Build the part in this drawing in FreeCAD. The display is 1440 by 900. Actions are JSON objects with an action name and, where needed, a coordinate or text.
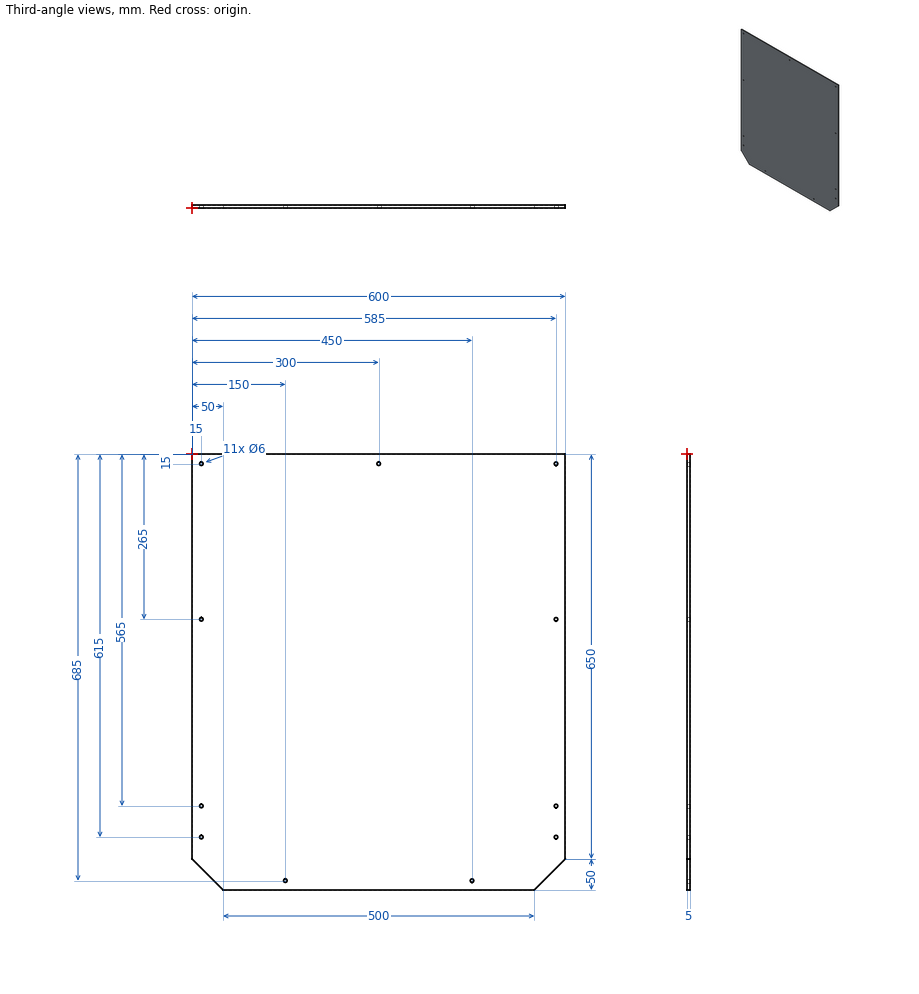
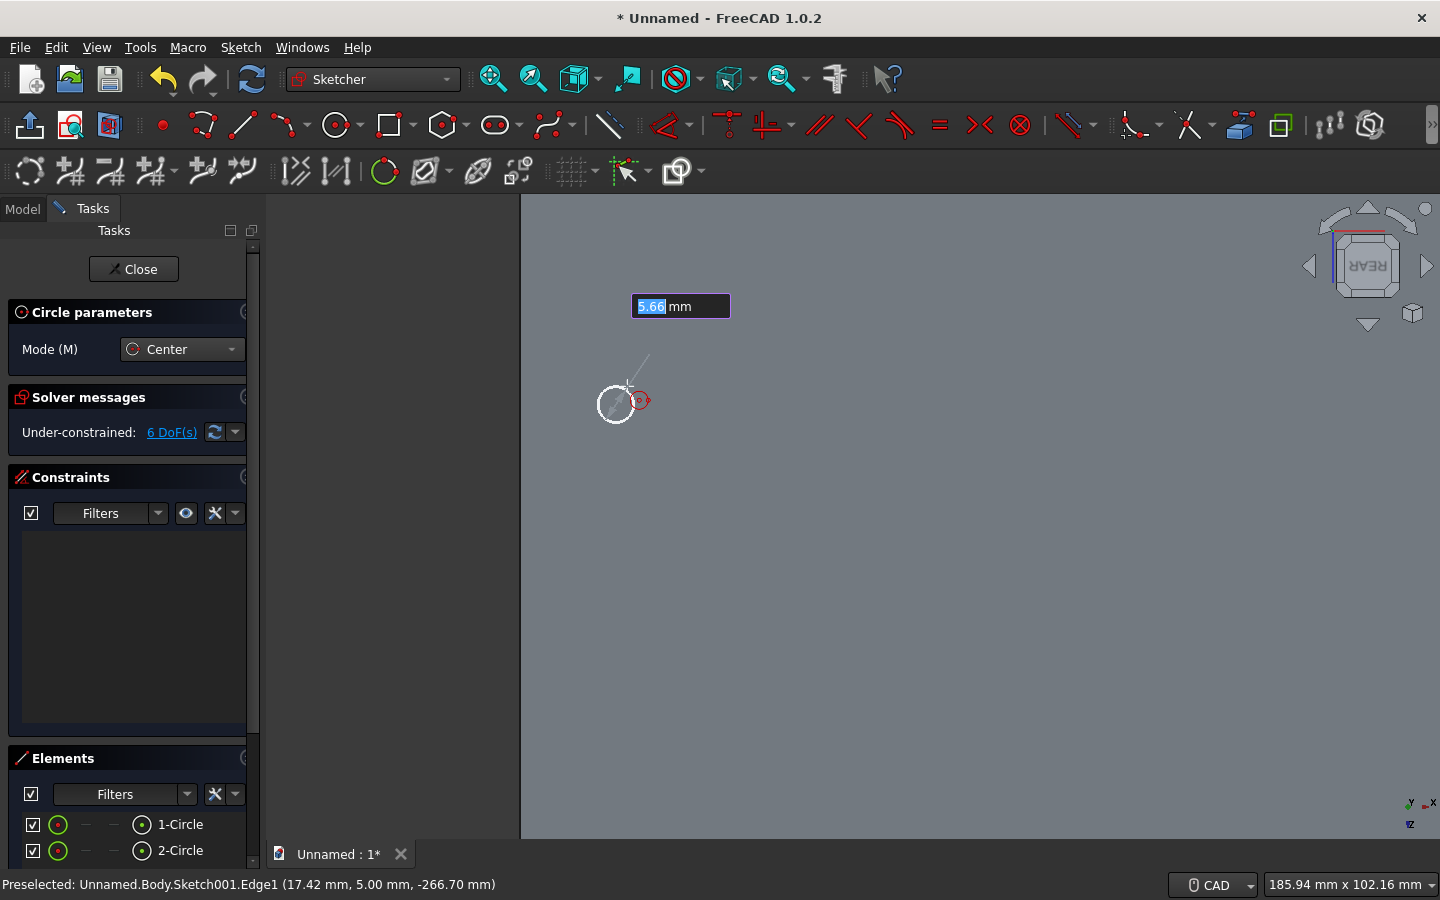
{"action": "left_click", "coordinate": [628, 387]}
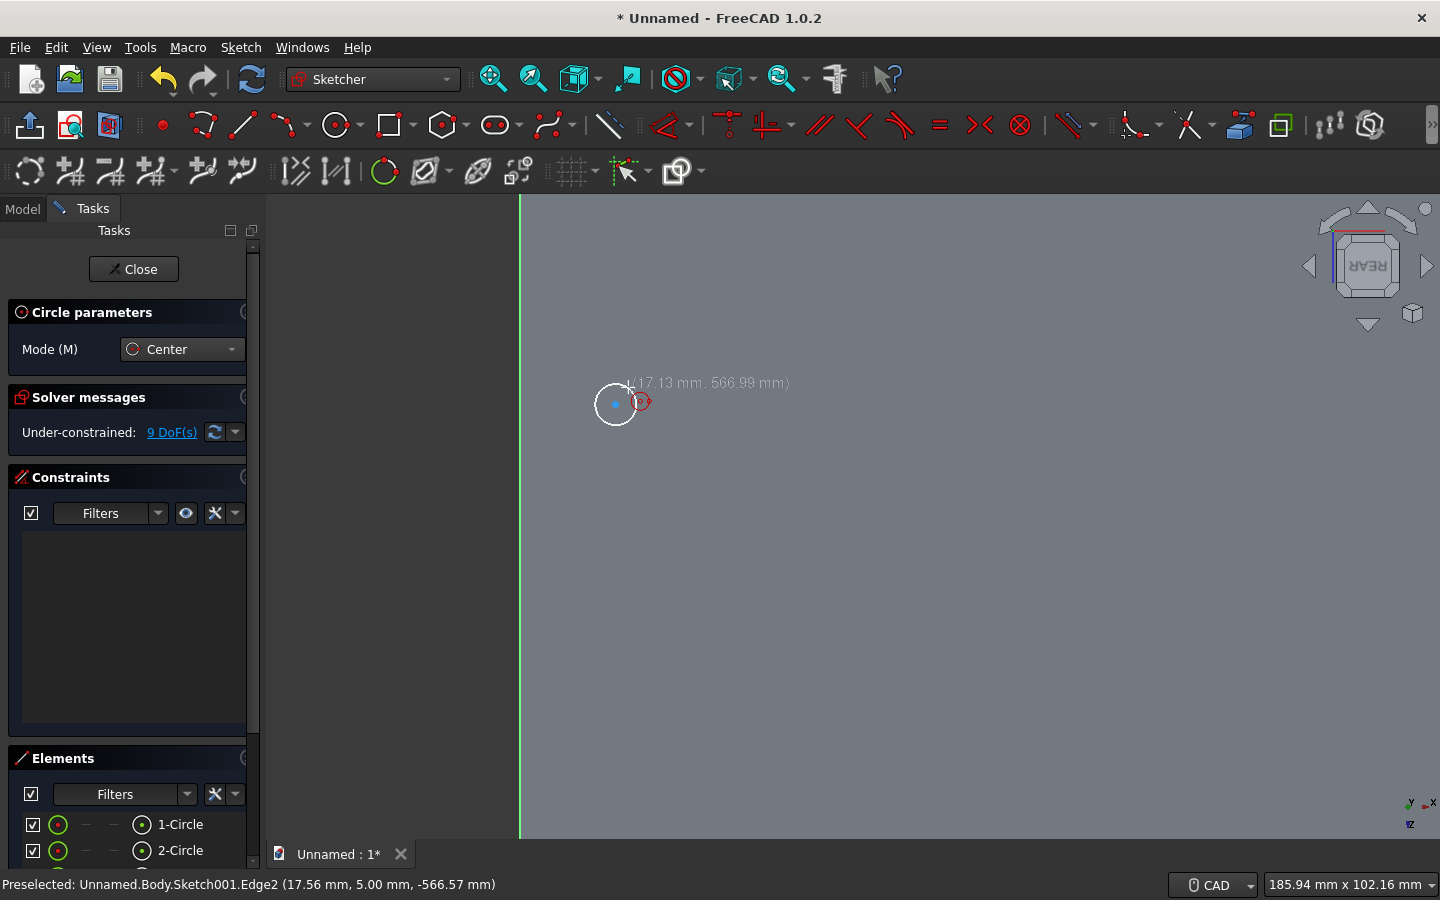
{"action": "scroll", "coordinate": [626, 389], "scroll_direction": "down", "scroll_amount": 12}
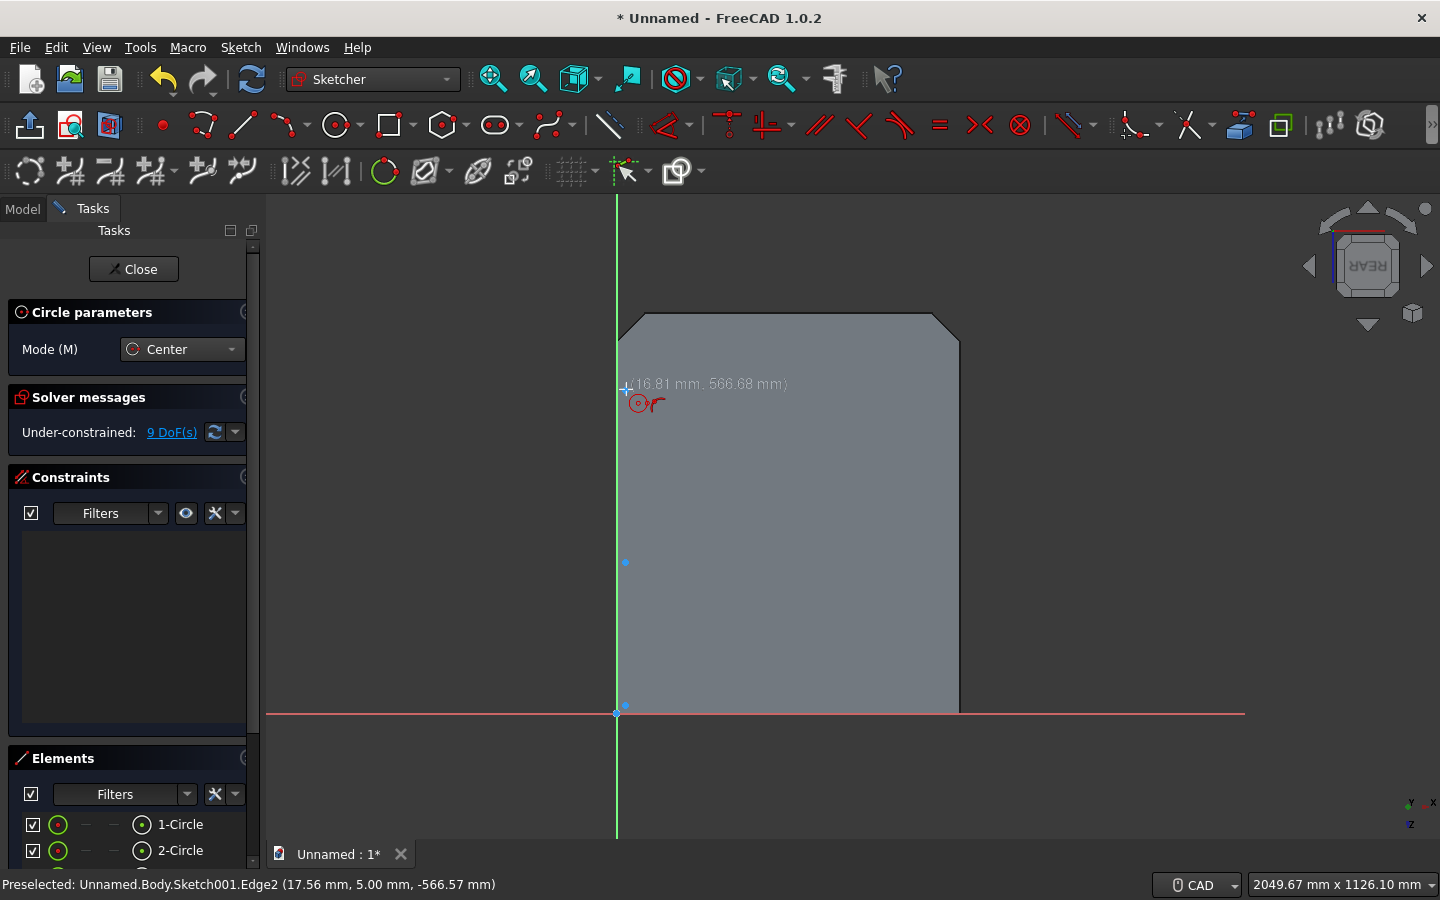
{"action": "scroll", "coordinate": [625, 362], "scroll_direction": "up", "scroll_amount": 13}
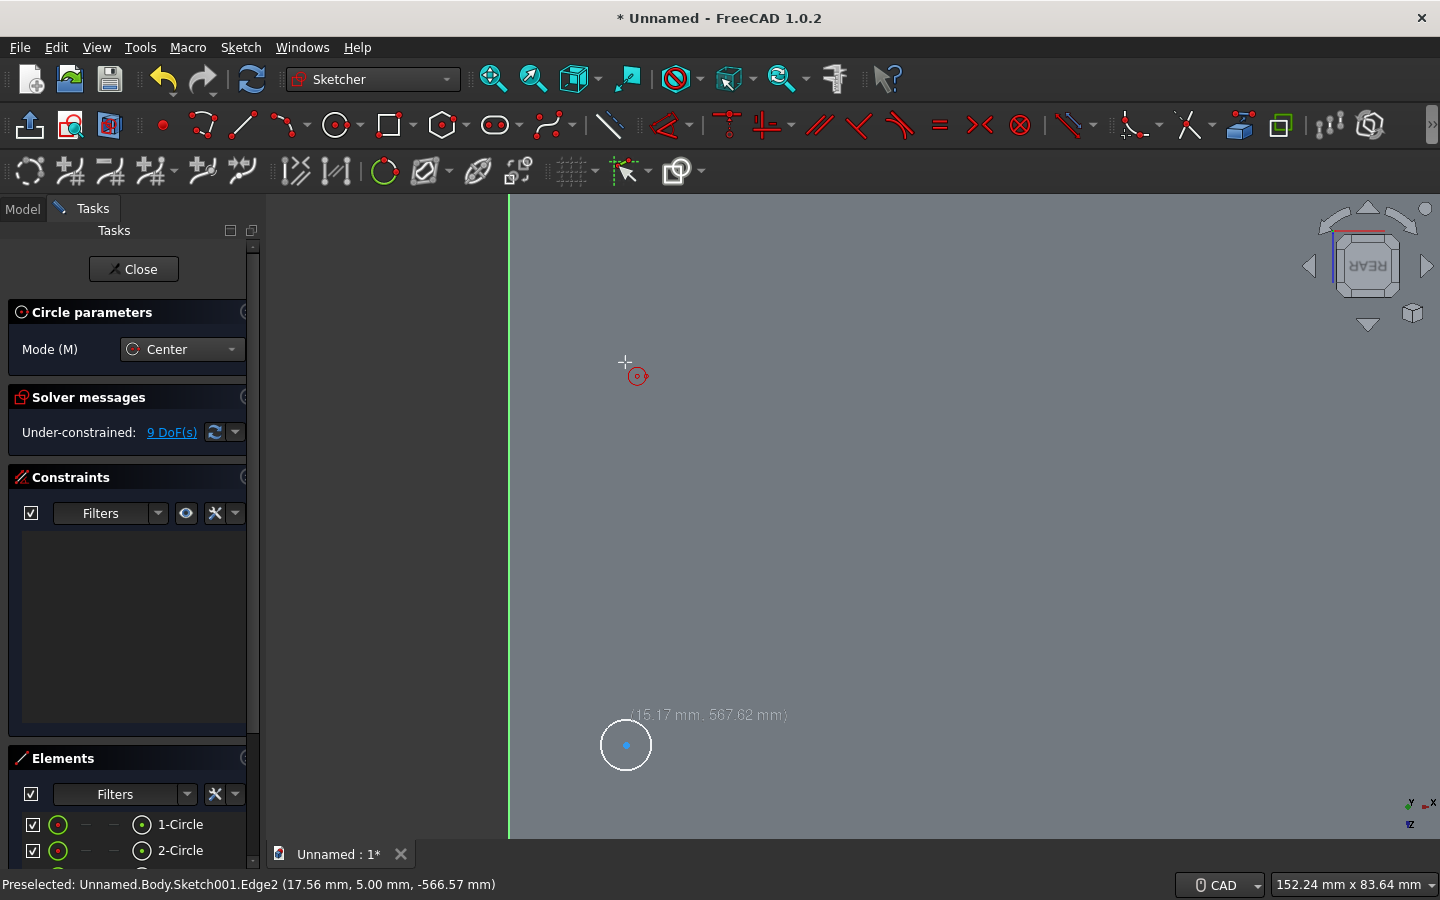
{"action": "scroll", "coordinate": [625, 362], "scroll_direction": "down", "scroll_amount": 13}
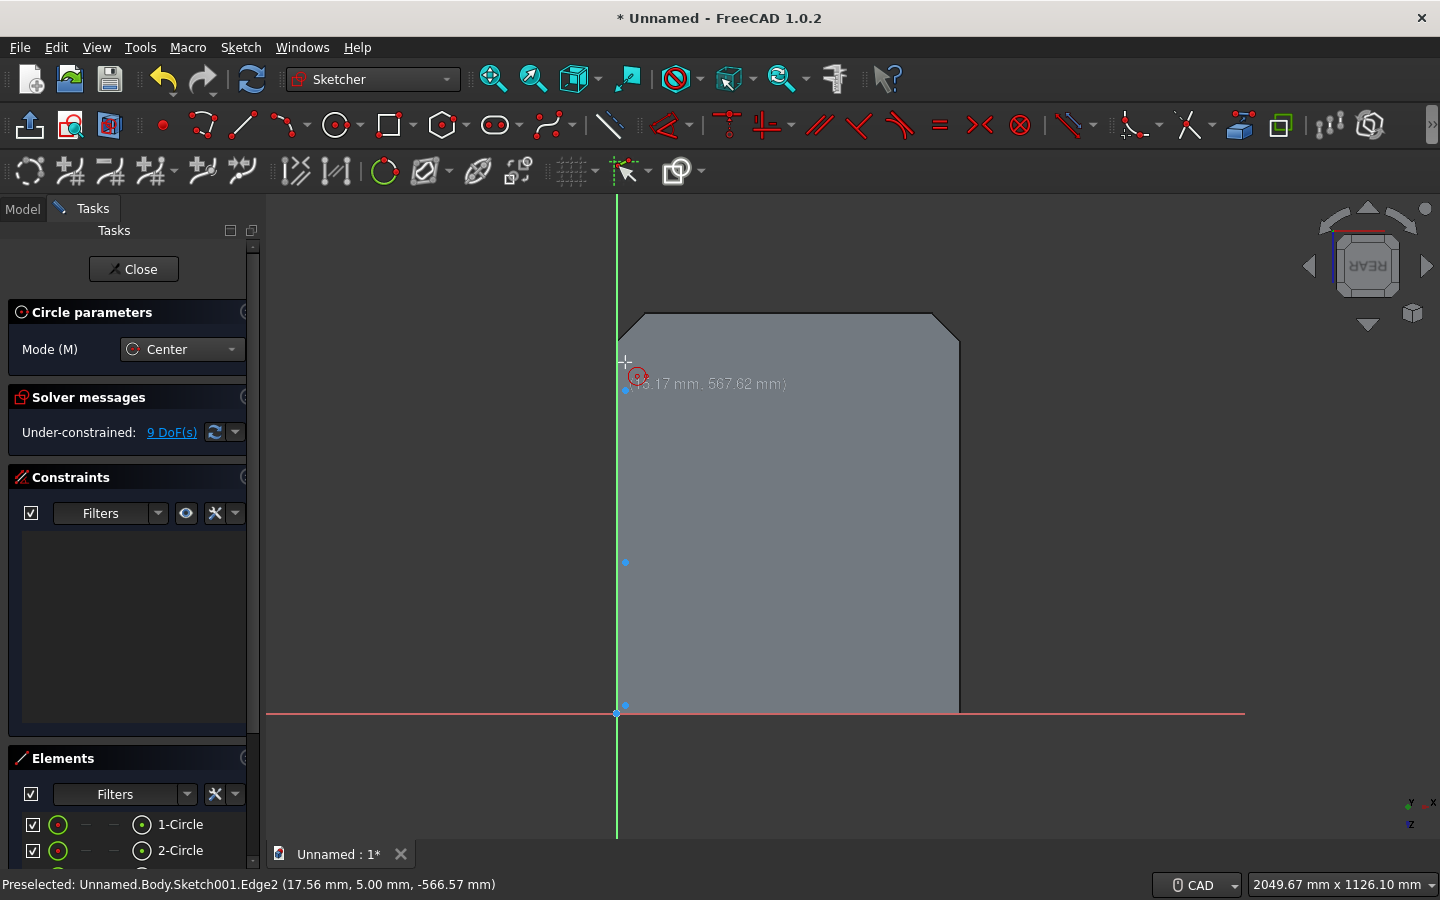
{"action": "scroll", "coordinate": [625, 362], "scroll_direction": "up", "scroll_amount": 4}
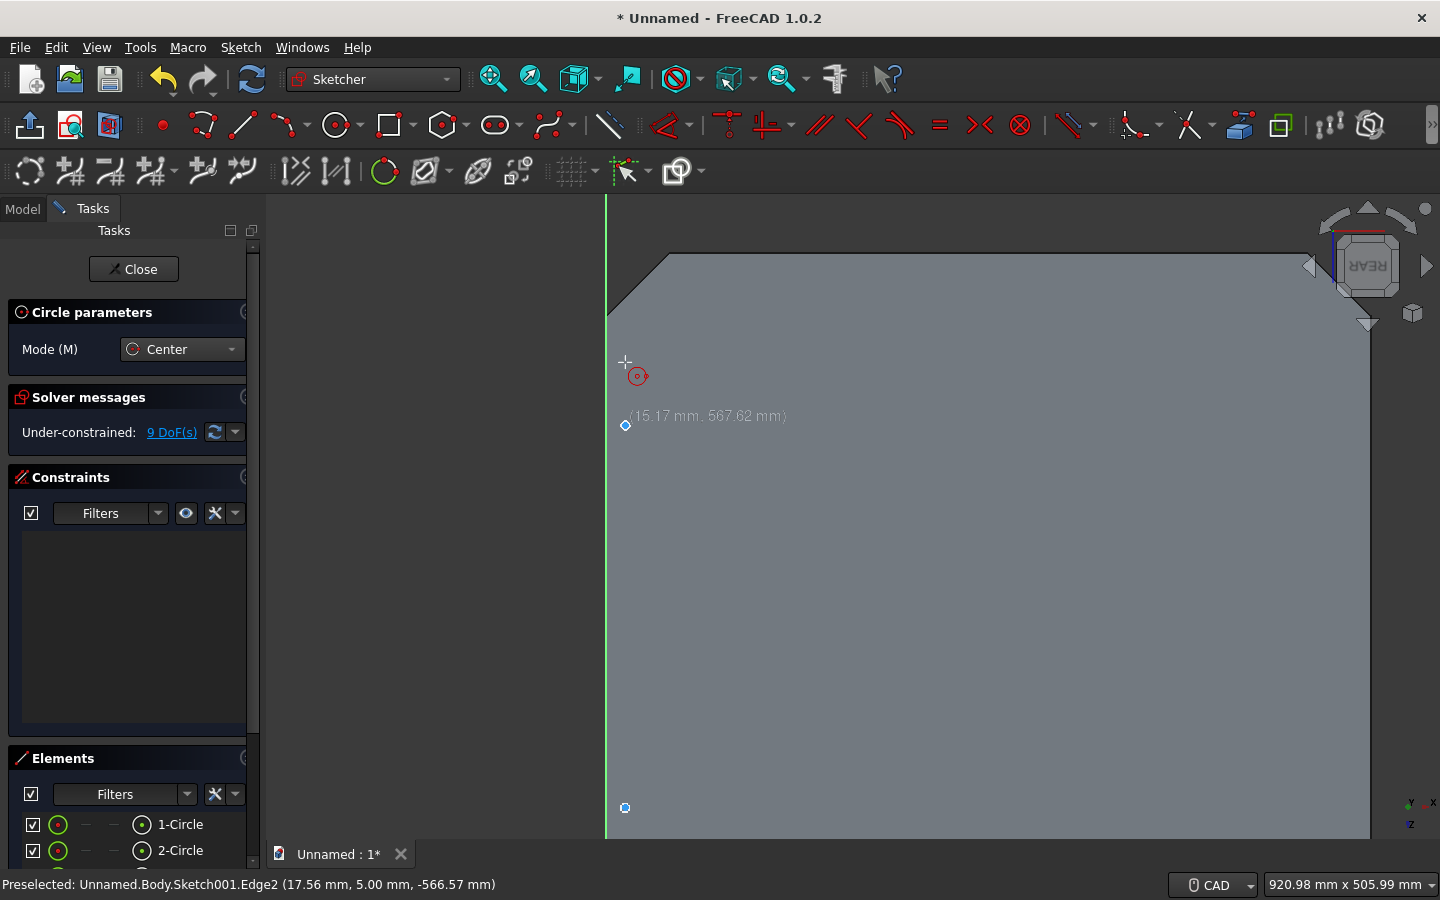
{"action": "left_click", "coordinate": [625, 361]}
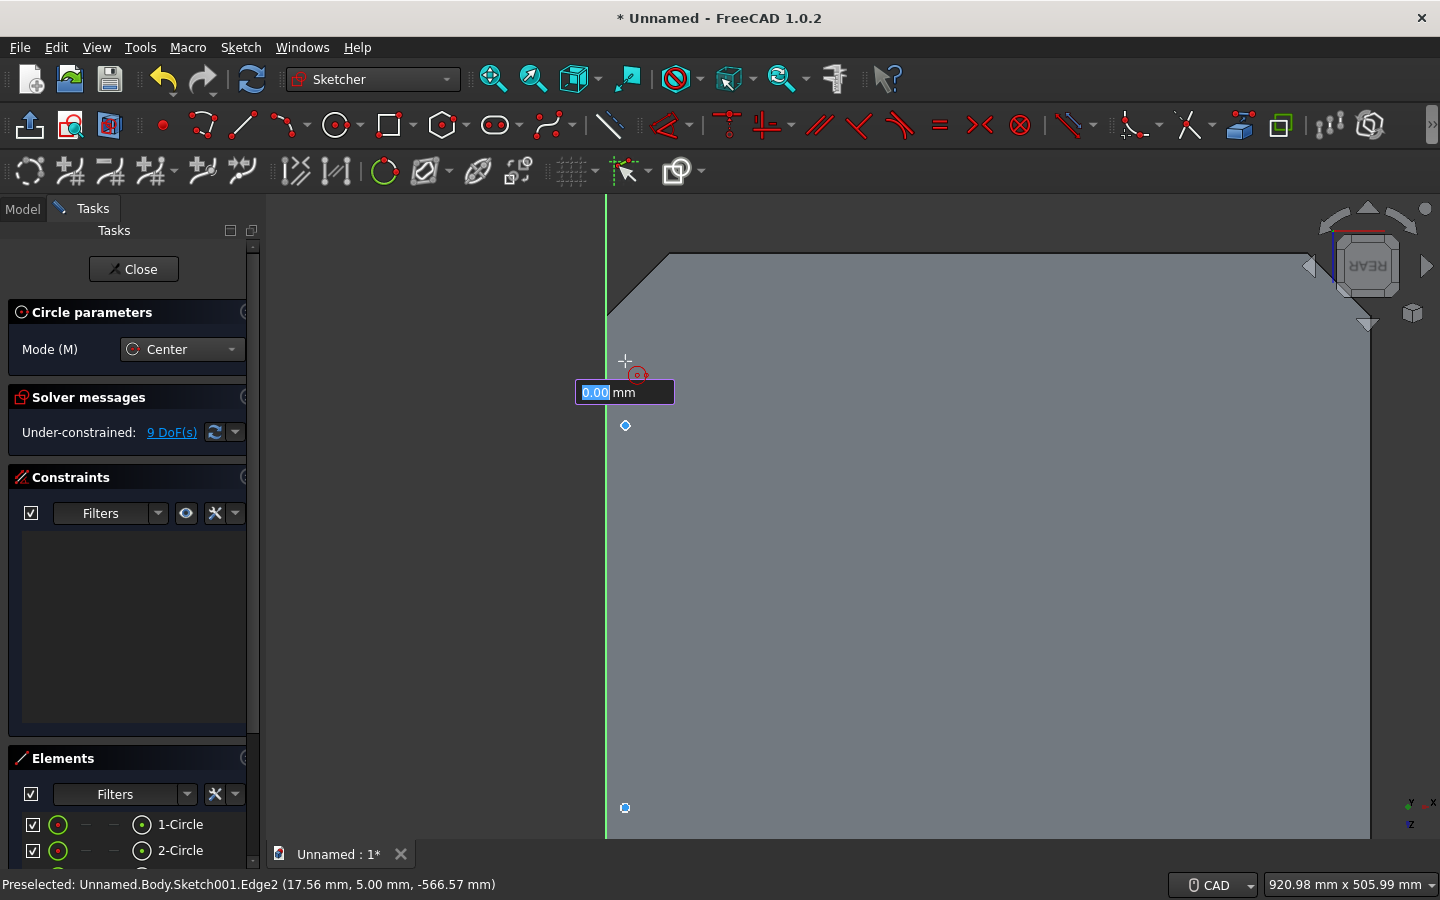
{"action": "scroll", "coordinate": [628, 358], "scroll_direction": "up", "scroll_amount": 8}